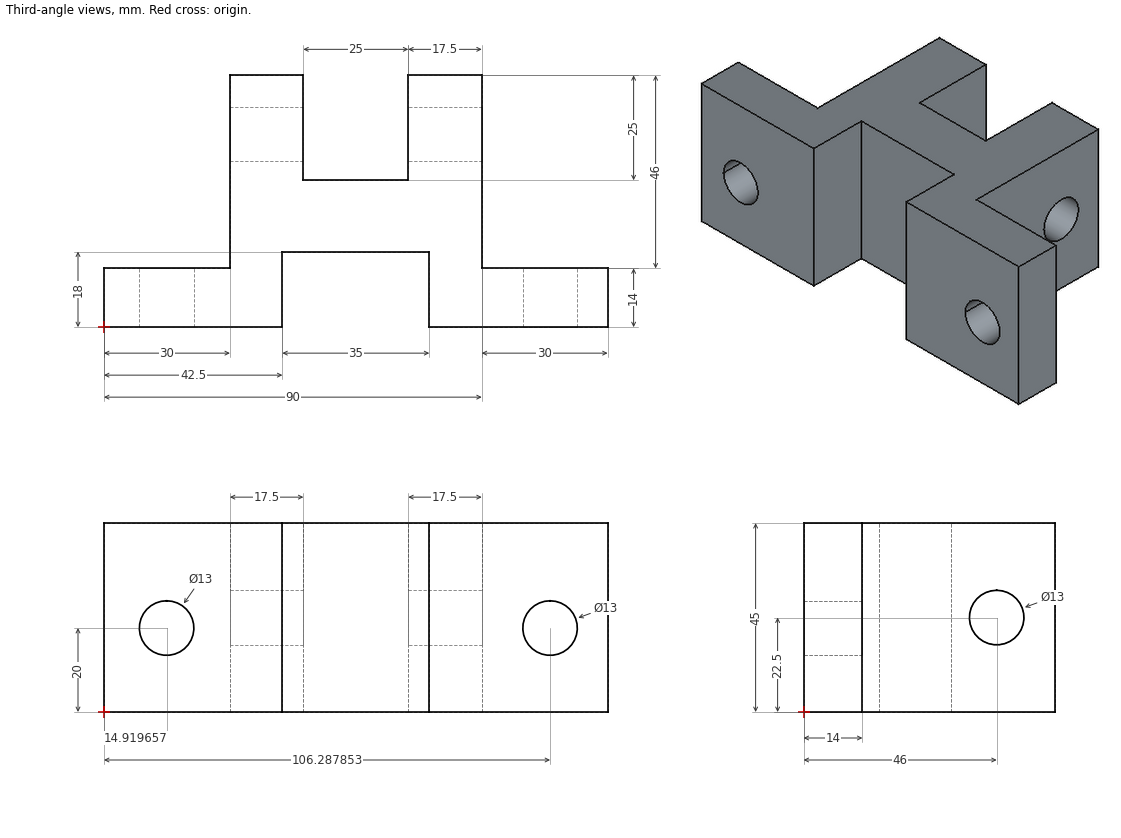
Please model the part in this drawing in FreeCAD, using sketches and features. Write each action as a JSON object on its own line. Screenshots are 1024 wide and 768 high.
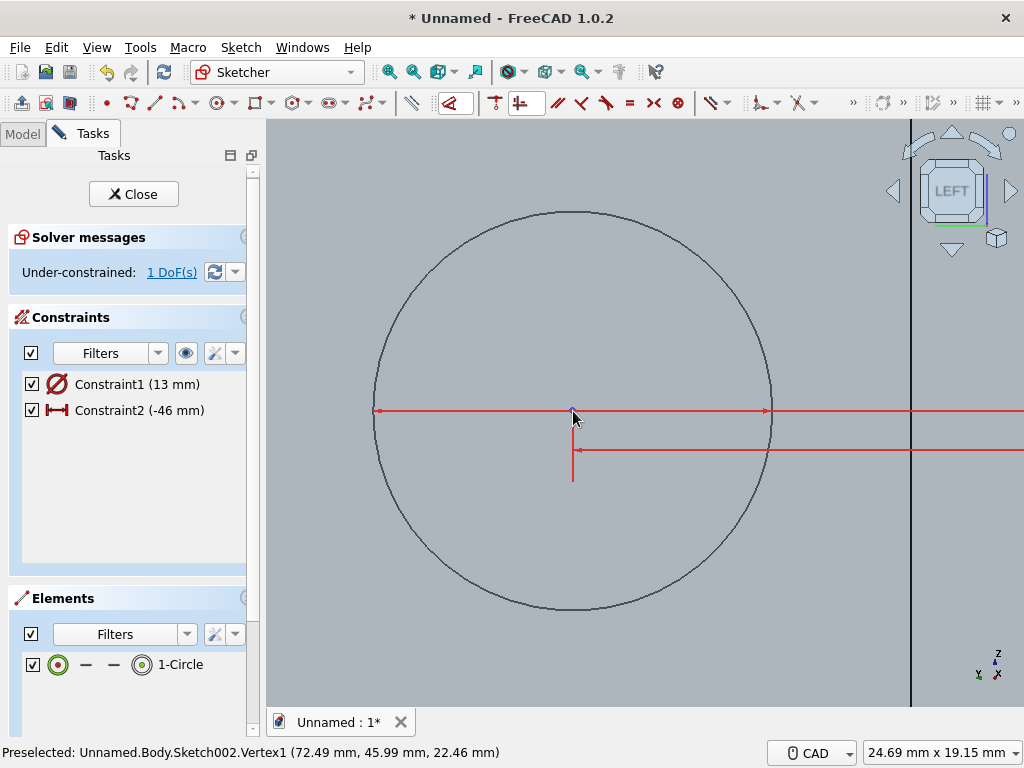
{"action": "left_click", "coordinate": [573, 411]}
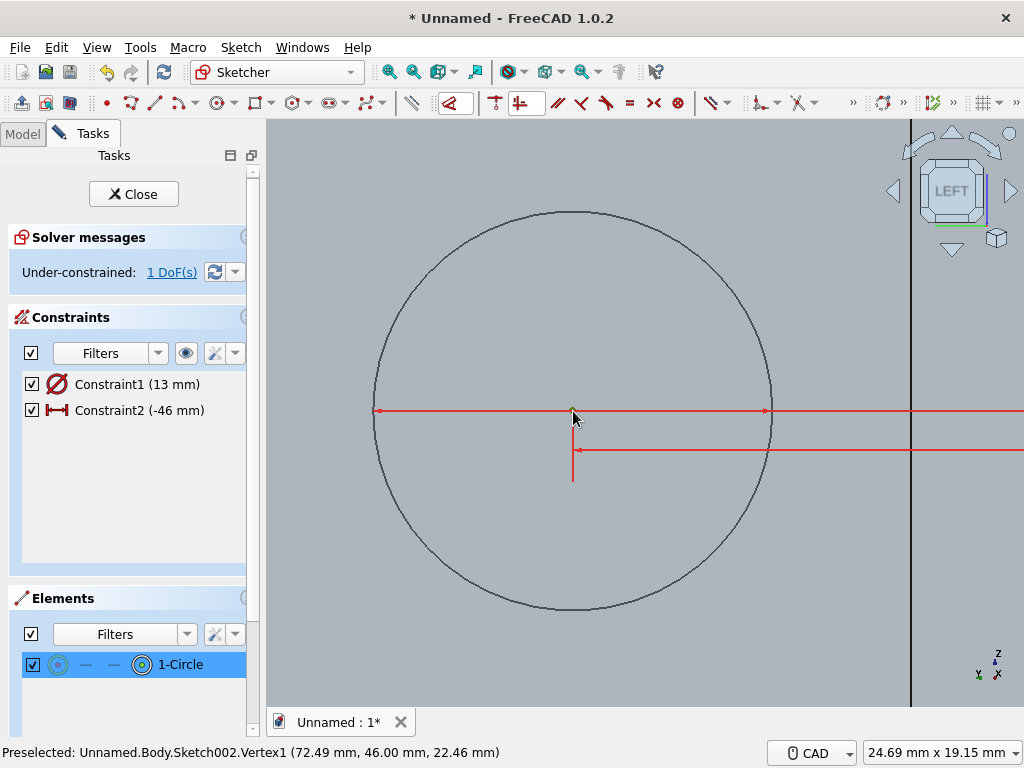
{"action": "key", "text": "i"}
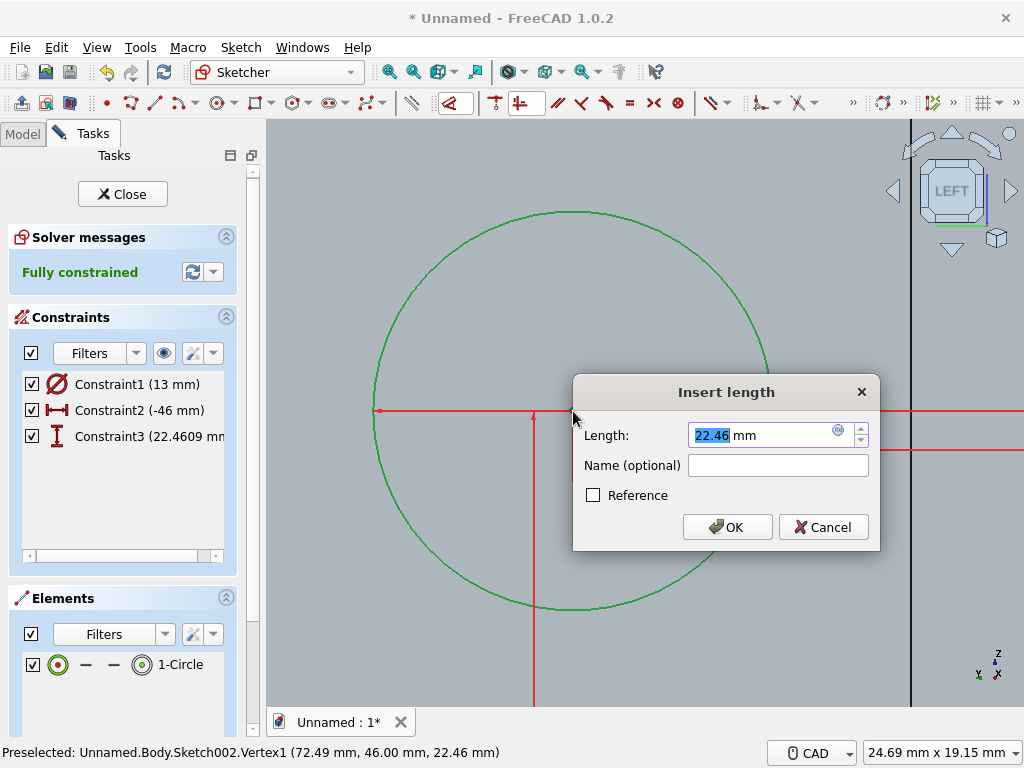
{"action": "type", "text": "22.5"}
{"action": "key", "text": "Return"}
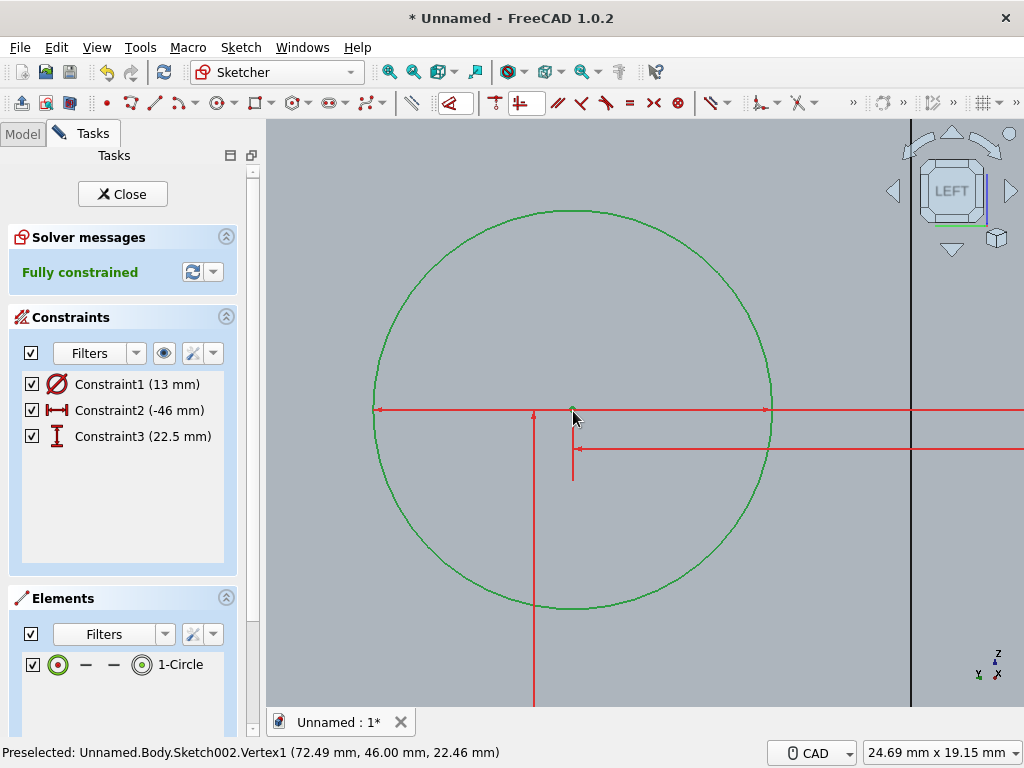
{"action": "left_click", "coordinate": [123, 194]}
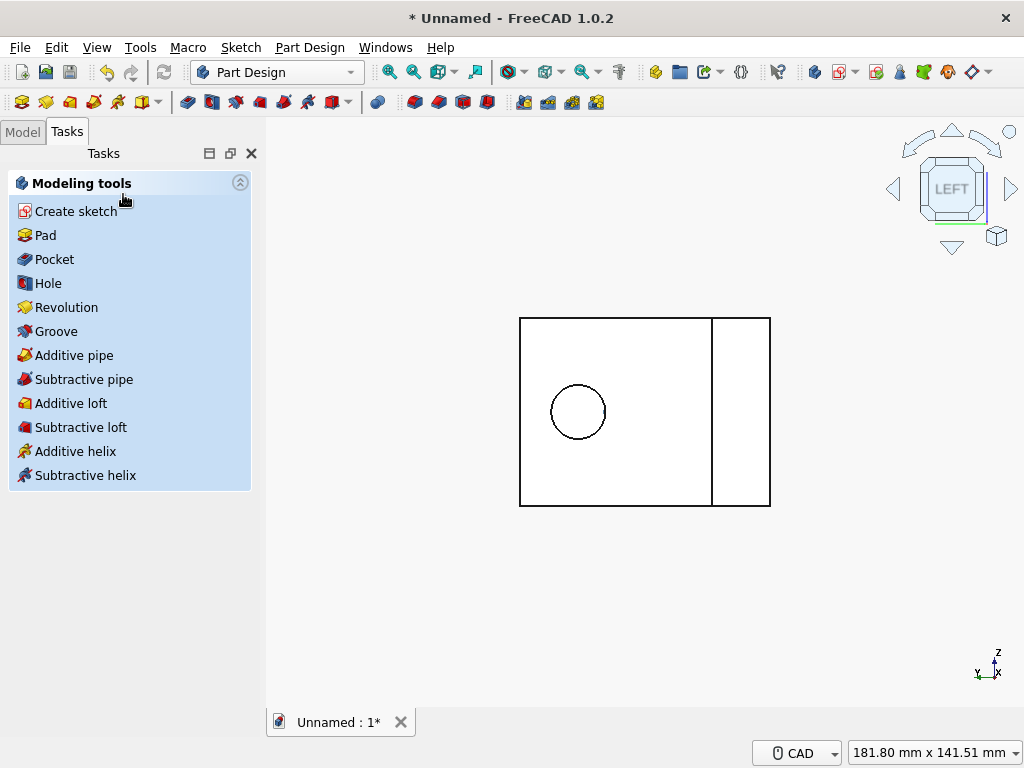
{"action": "left_click", "coordinate": [188, 102]}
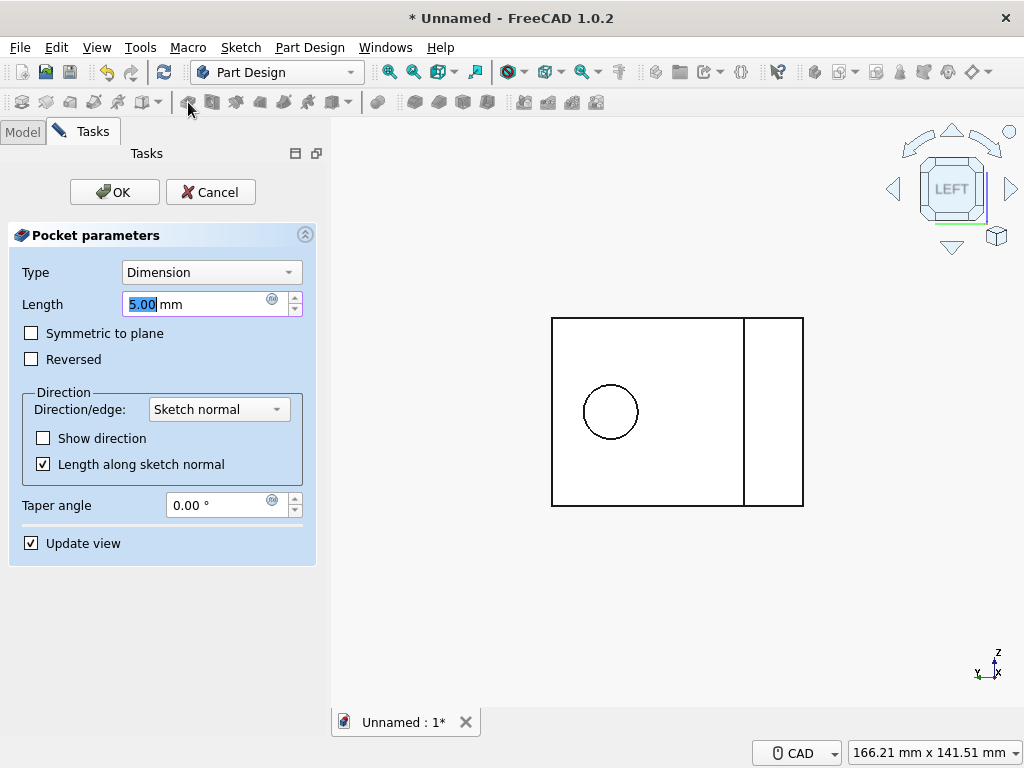
{"action": "type", "text": "17.5"}
{"action": "key", "text": "Tab"}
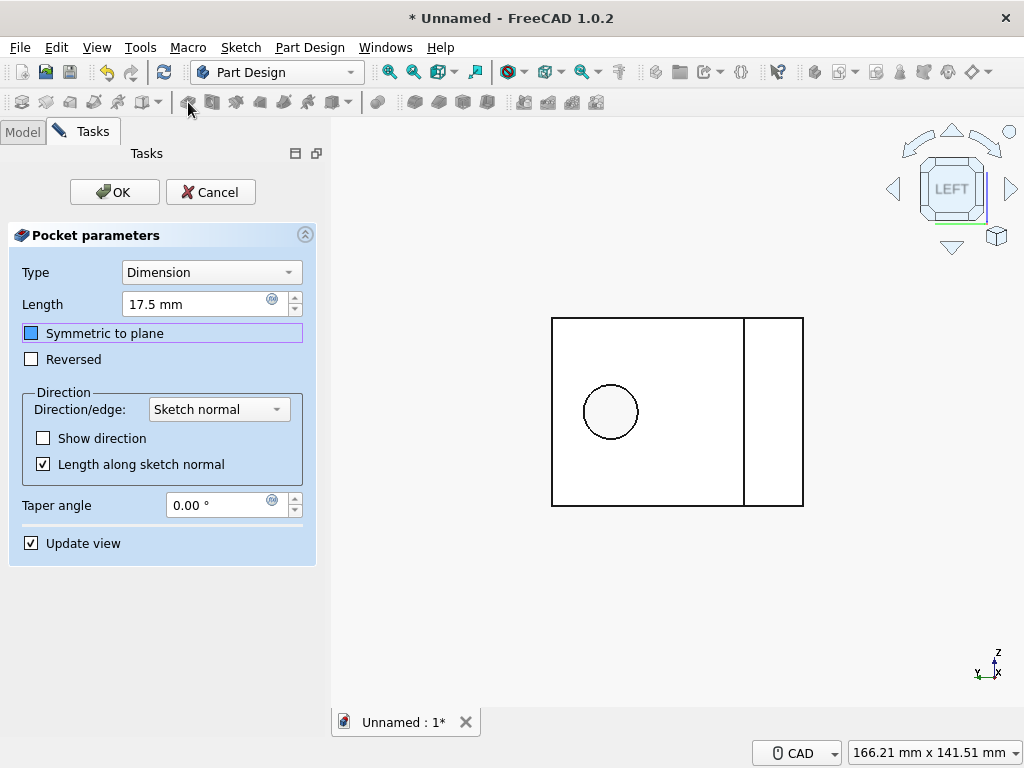
{"action": "left_click", "coordinate": [115, 192]}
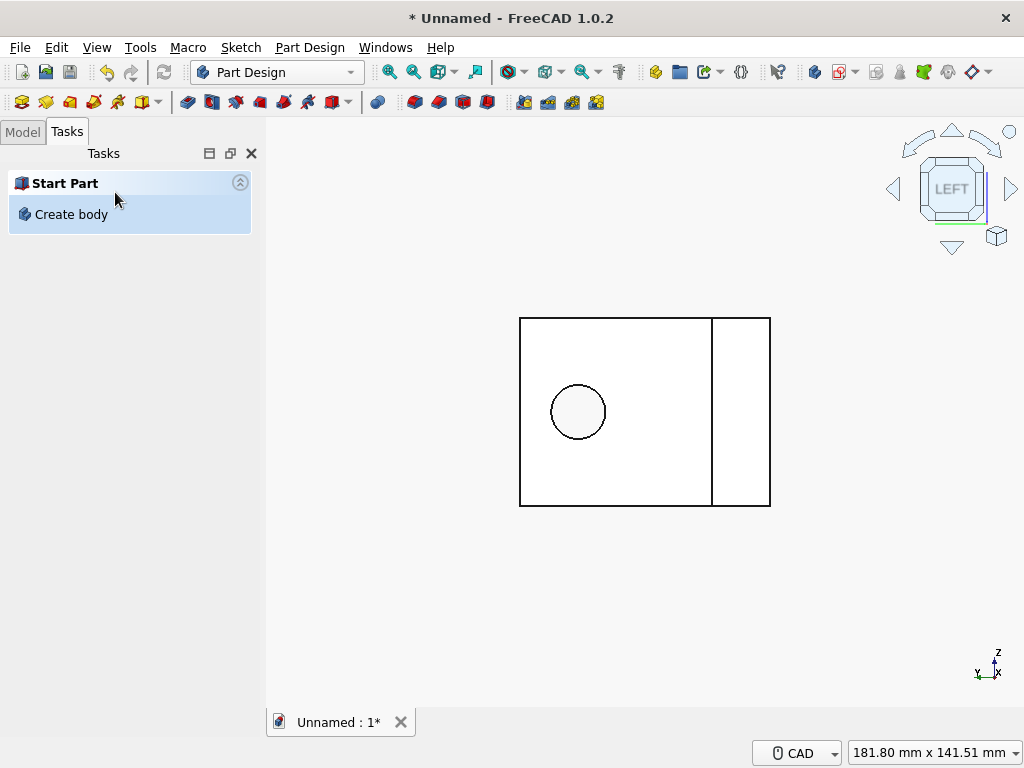
{"action": "left_click", "coordinate": [390, 72]}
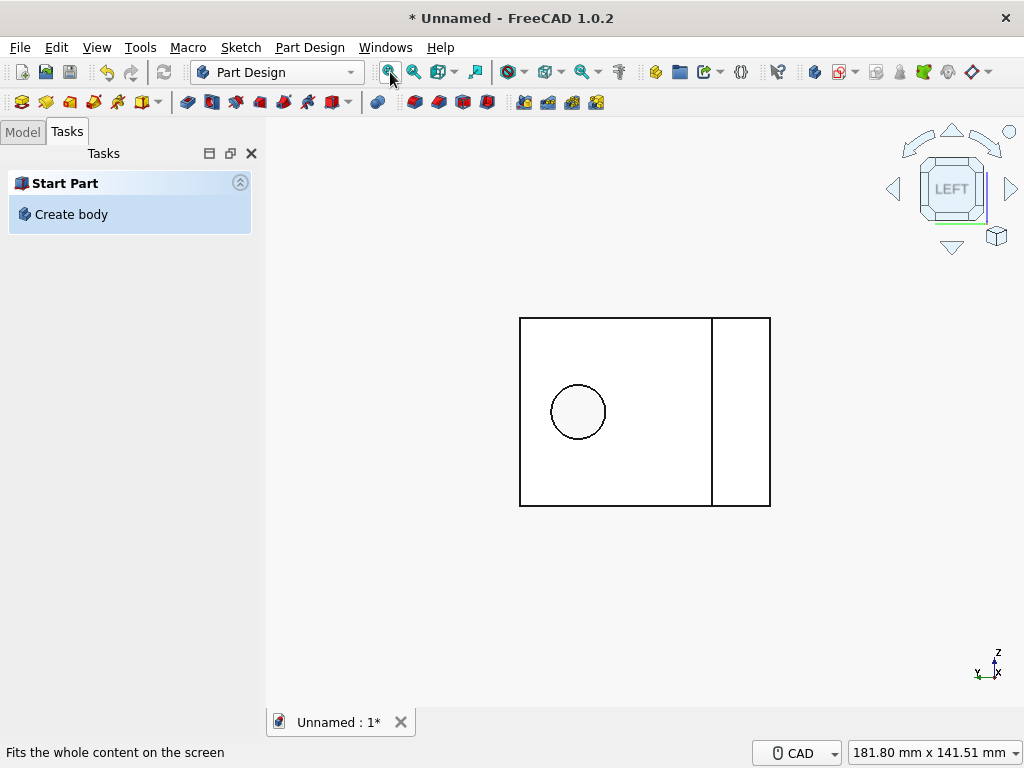
{"action": "key", "text": "4"}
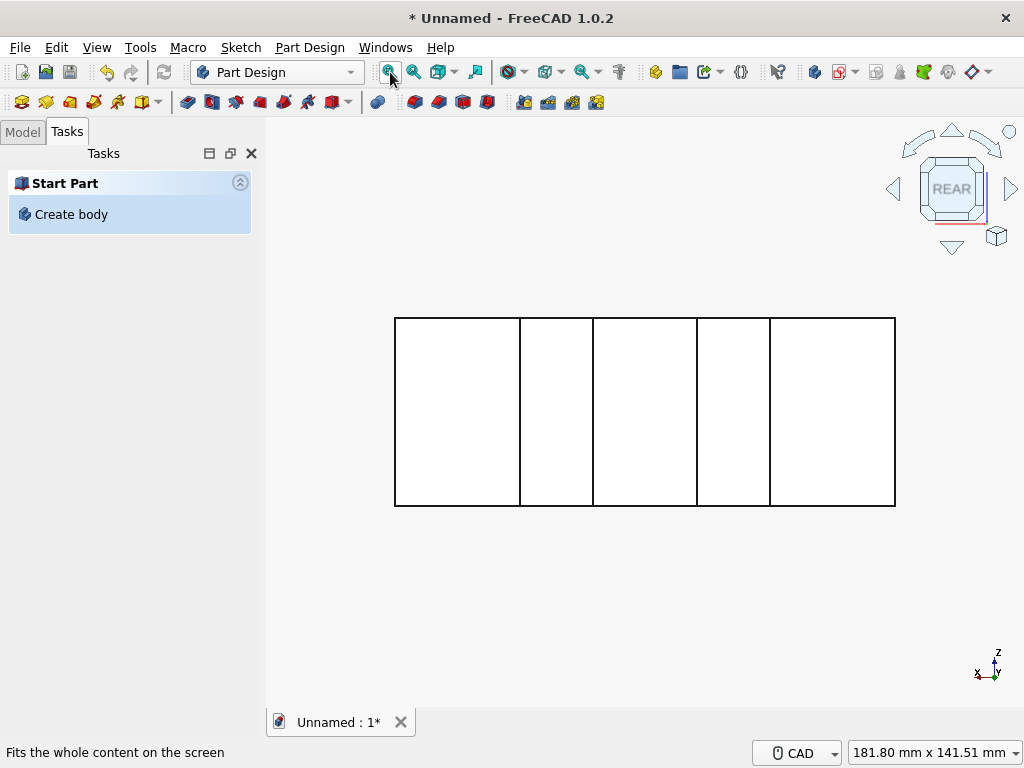
{"action": "left_click", "coordinate": [833, 384]}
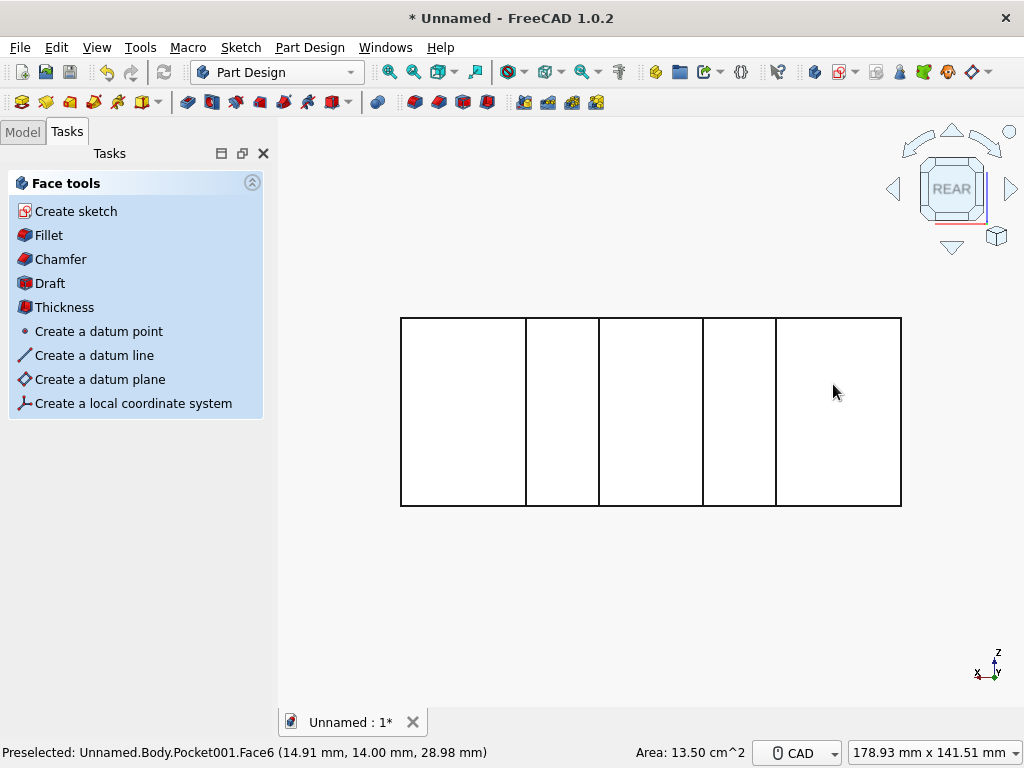
{"action": "left_click", "coordinate": [840, 72]}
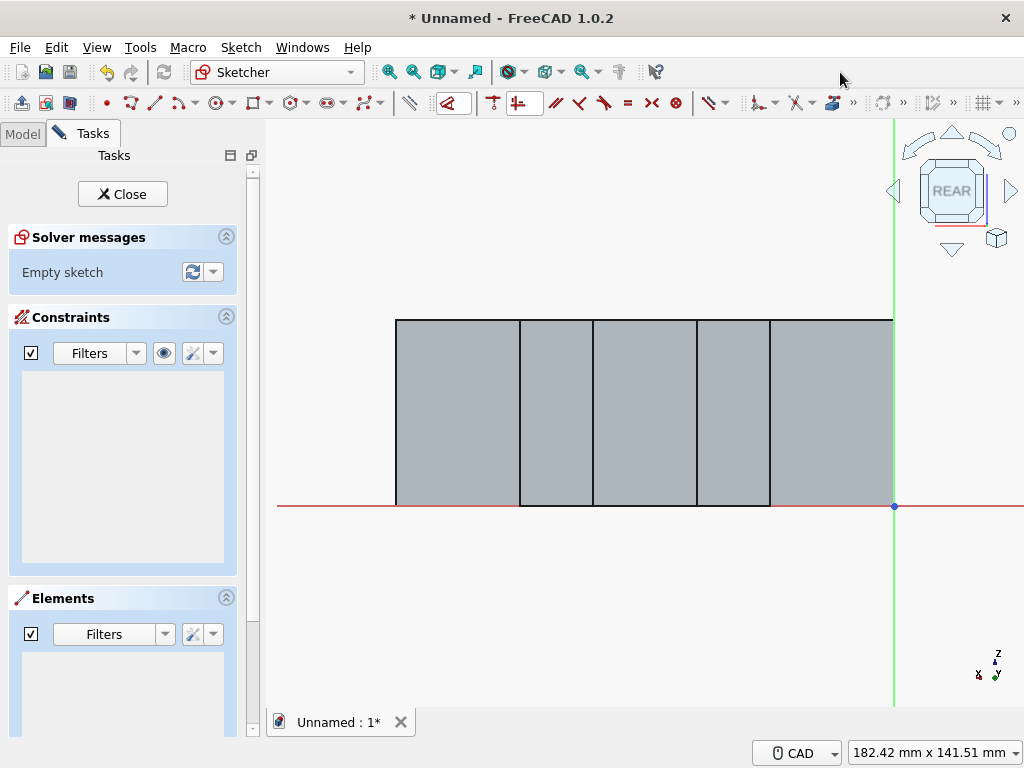
{"action": "left_click", "coordinate": [70, 104]}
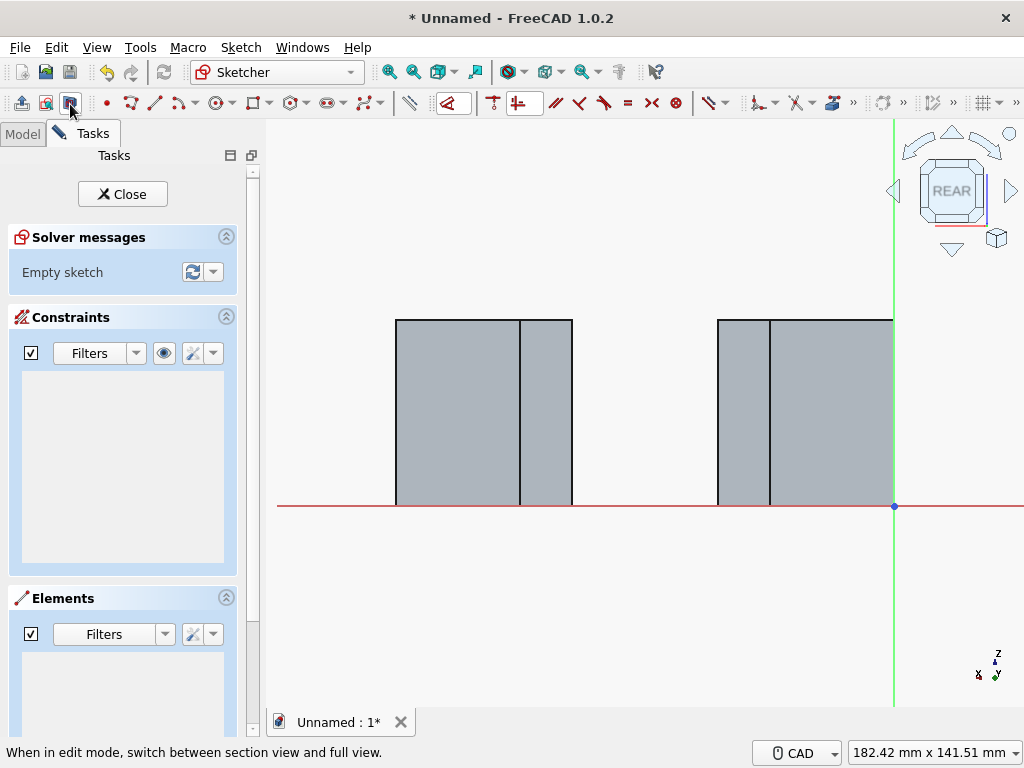
{"action": "scroll", "coordinate": [576, 413], "scroll_direction": "down", "scroll_amount": 5}